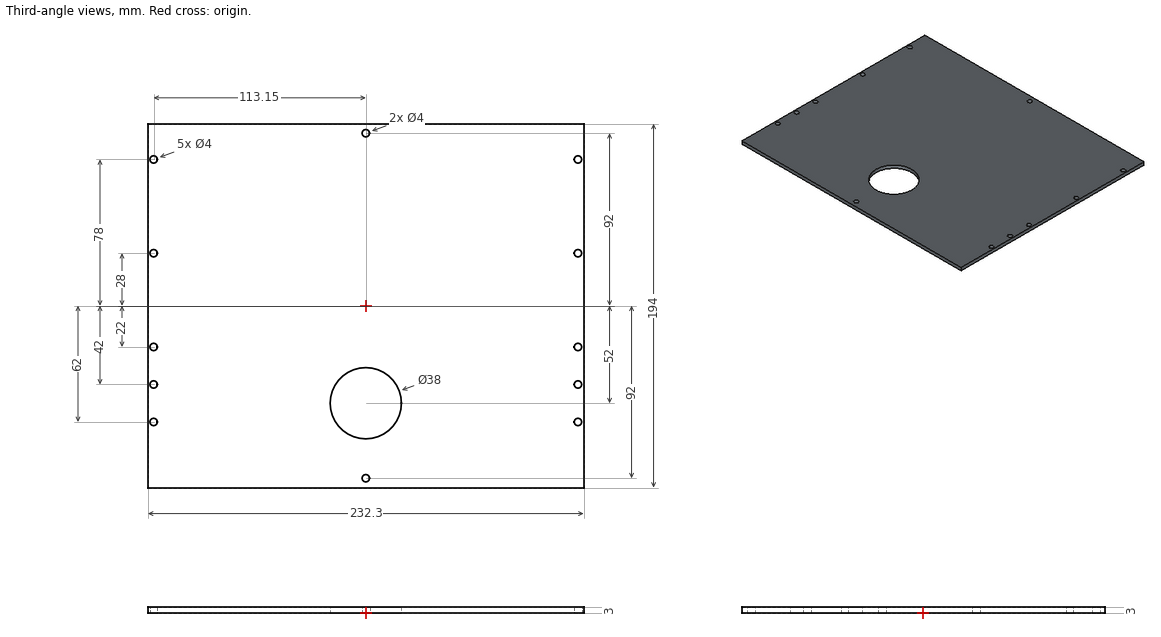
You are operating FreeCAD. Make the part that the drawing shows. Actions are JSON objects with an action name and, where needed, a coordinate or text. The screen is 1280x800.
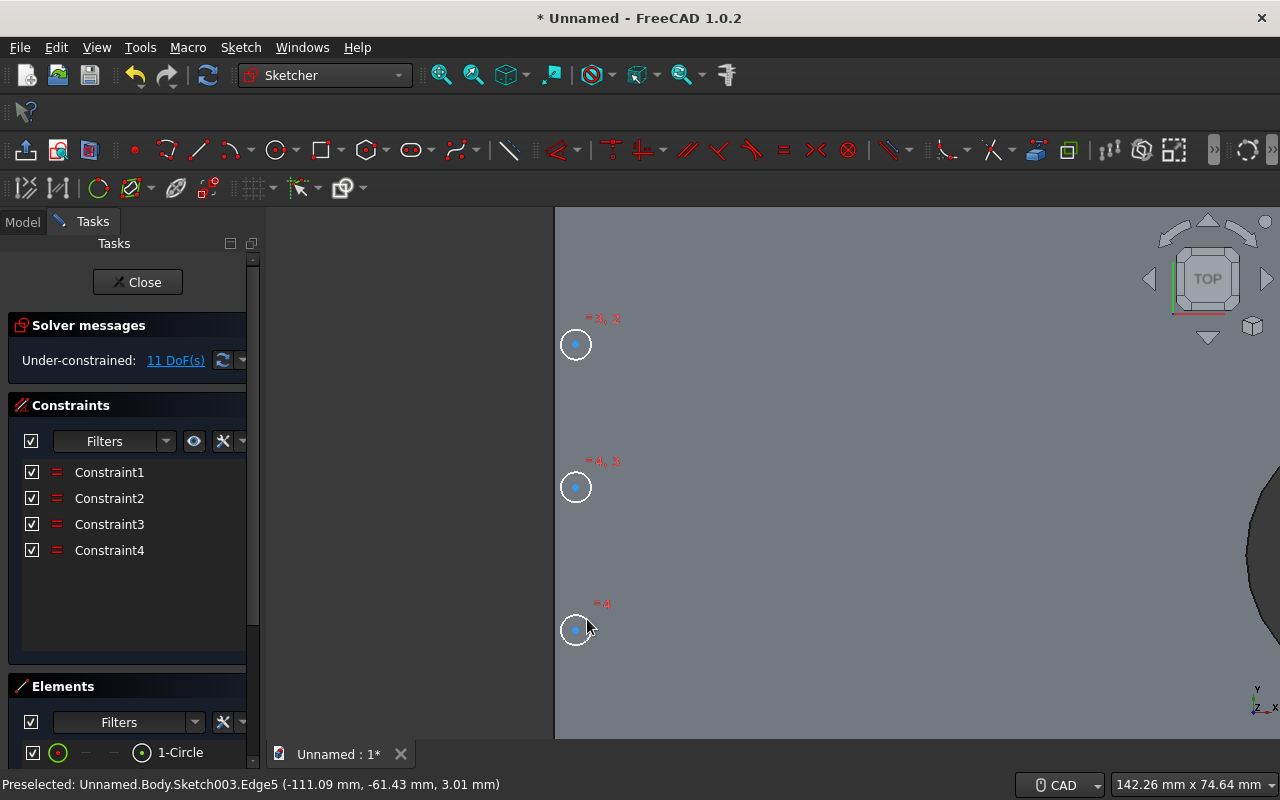
{"action": "scroll", "coordinate": [589, 622], "scroll_direction": "down", "scroll_amount": 6}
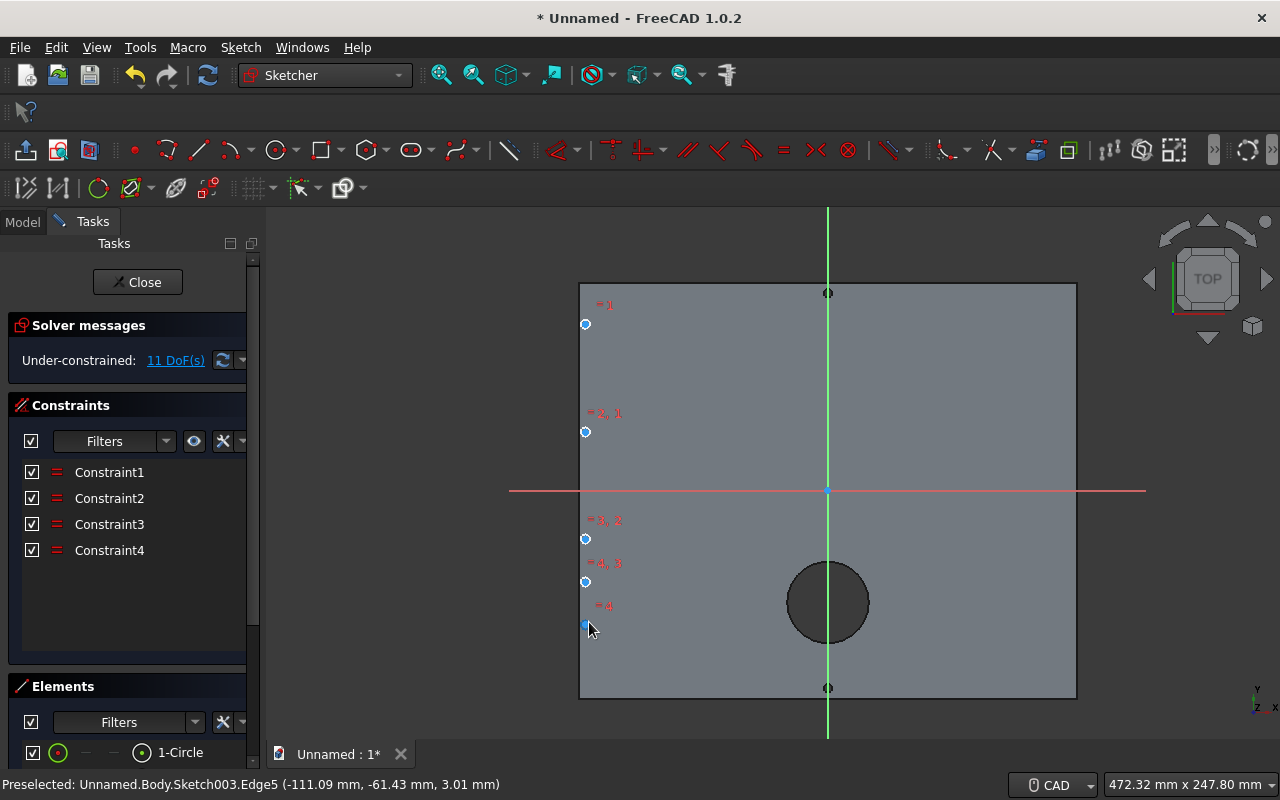
{"action": "left_click", "coordinate": [585, 324]}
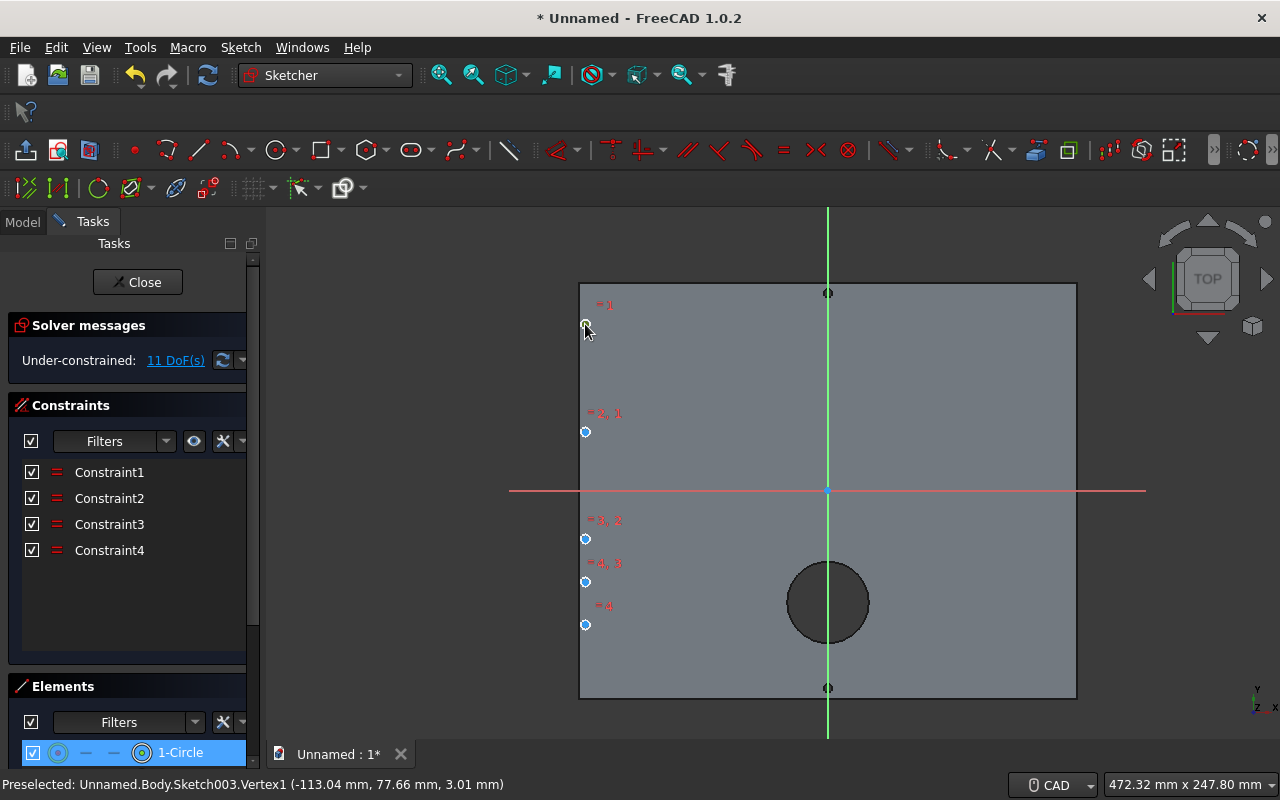
{"action": "left_click", "coordinate": [585, 432]}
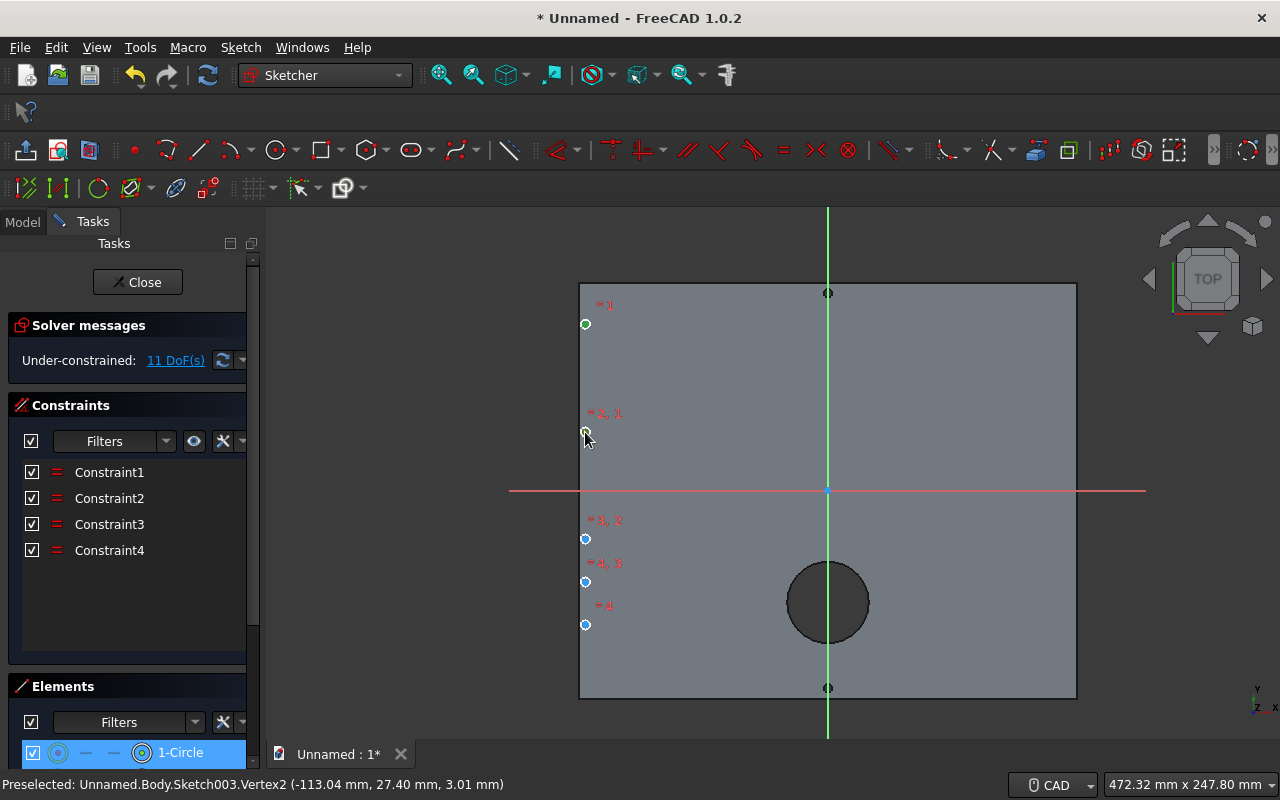
{"action": "key", "text": "v"}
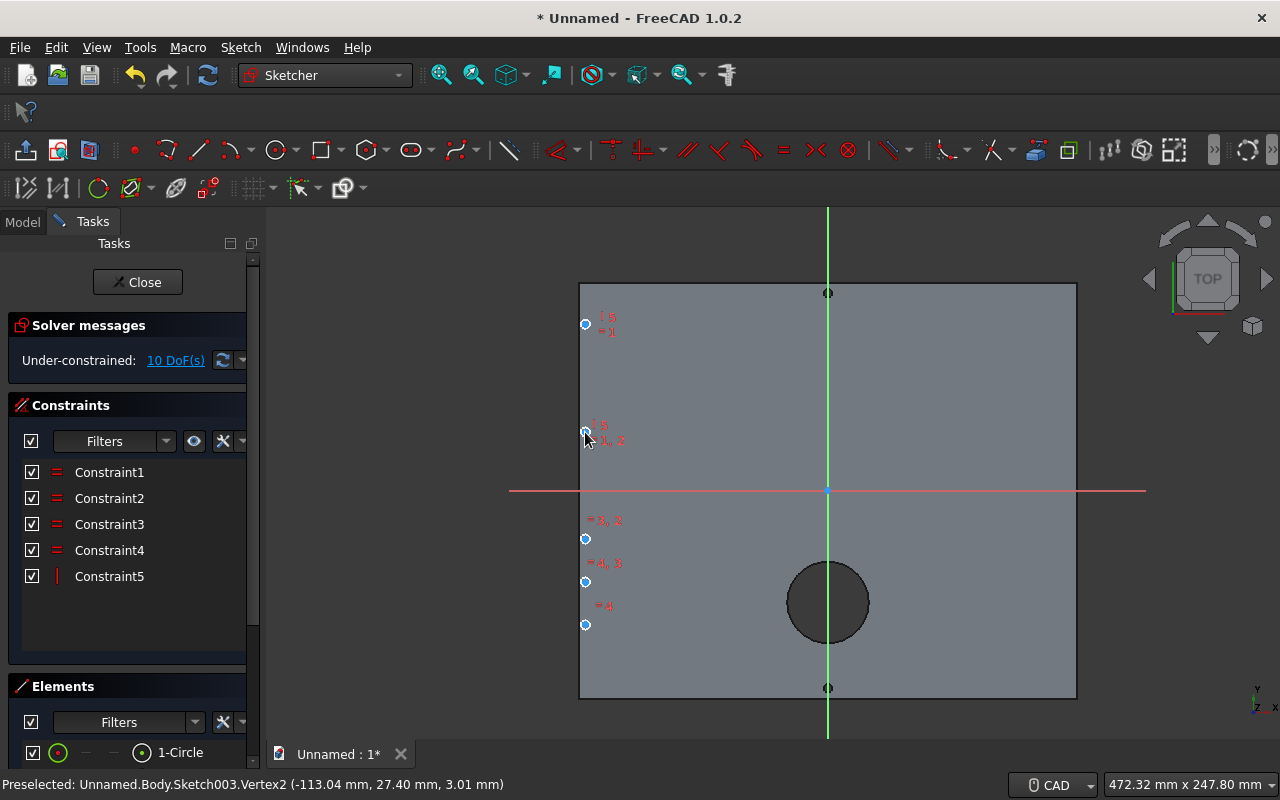
{"action": "left_click", "coordinate": [585, 432]}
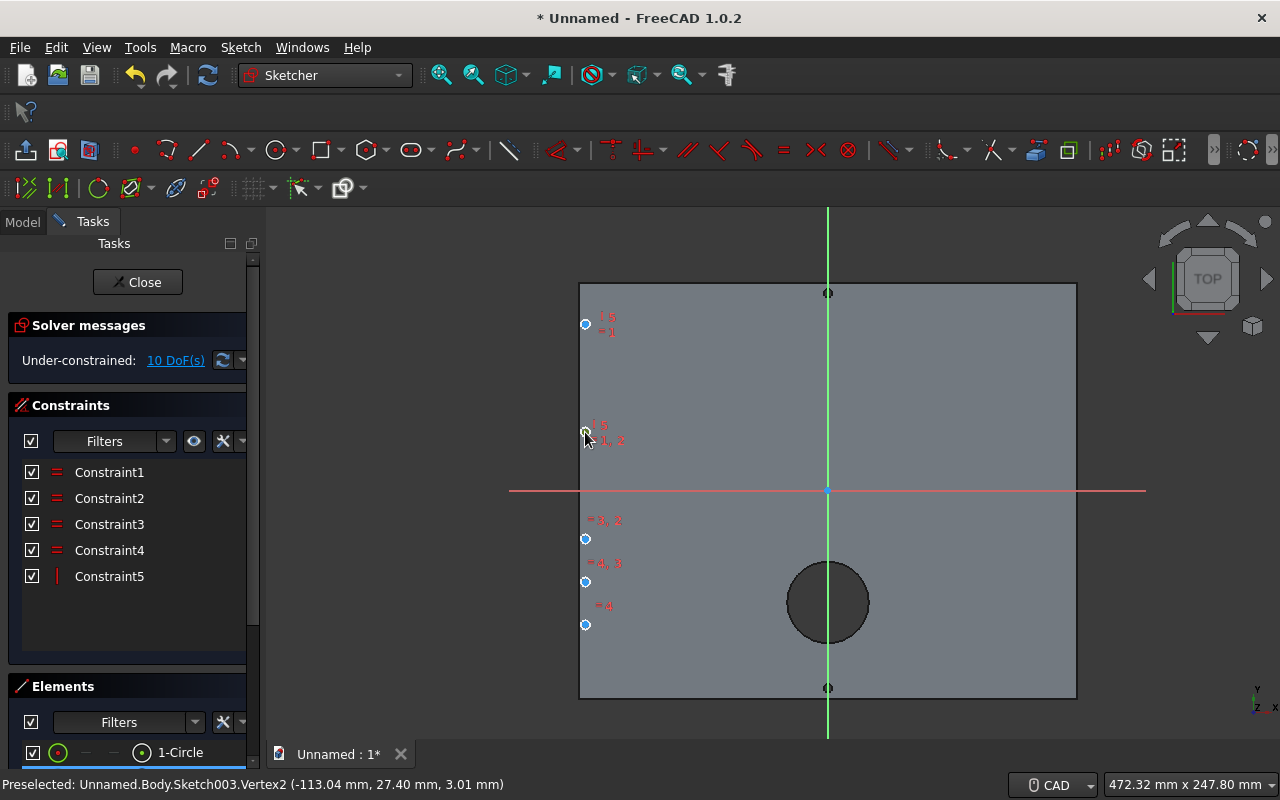
{"action": "left_click", "coordinate": [585, 539]}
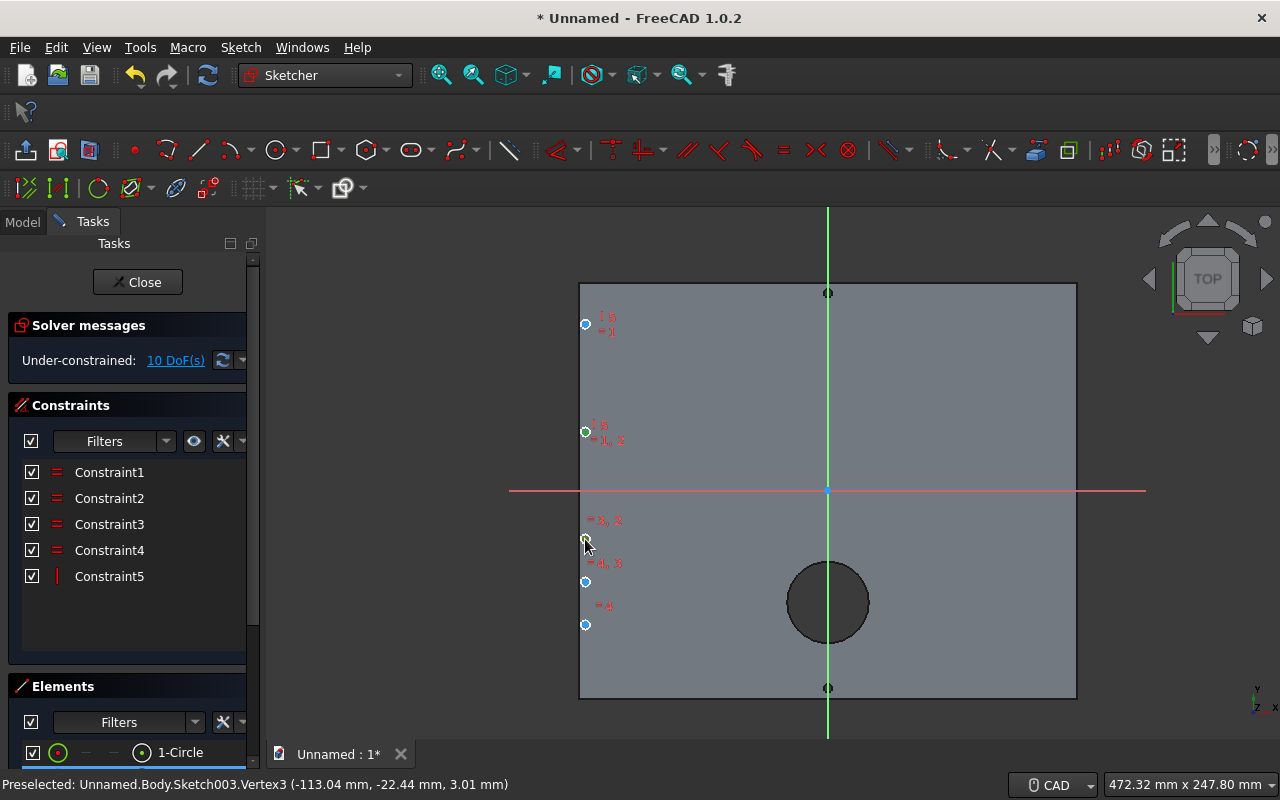
{"action": "key", "text": "v"}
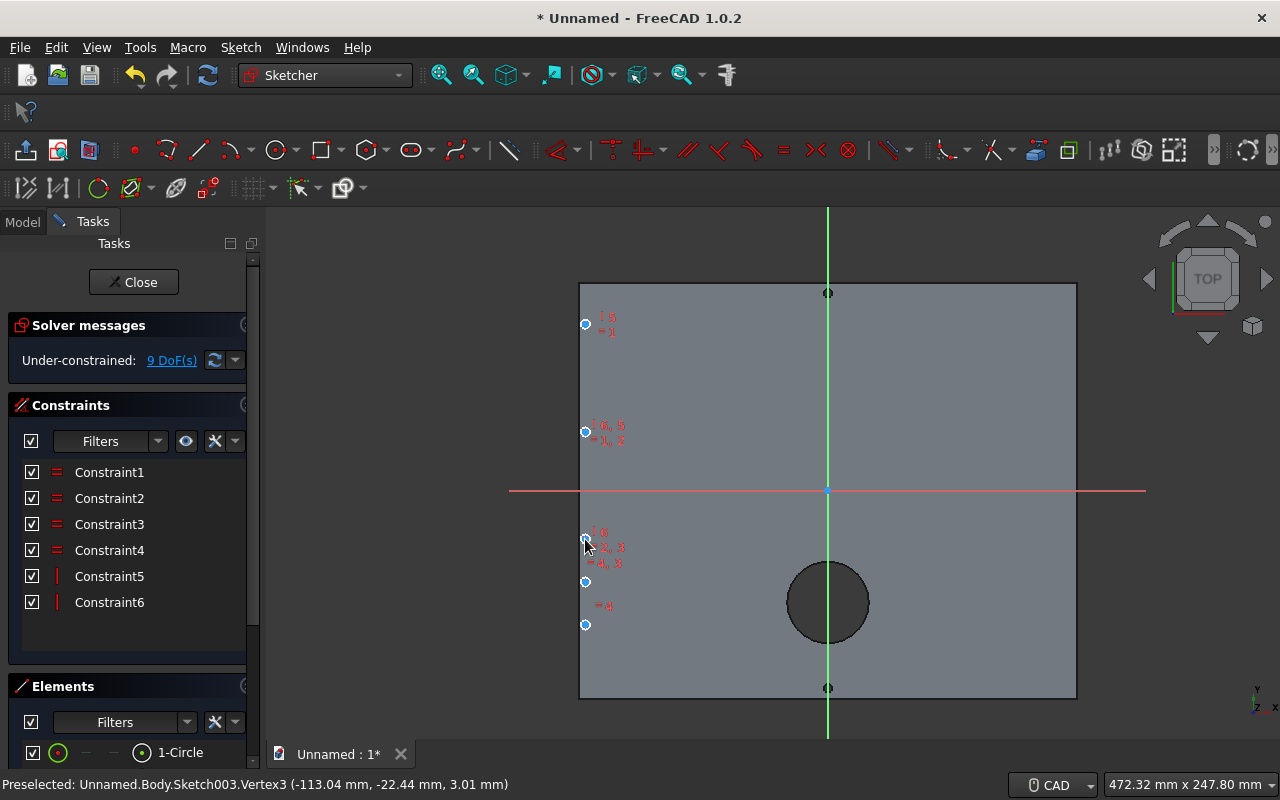
{"action": "left_click", "coordinate": [585, 539]}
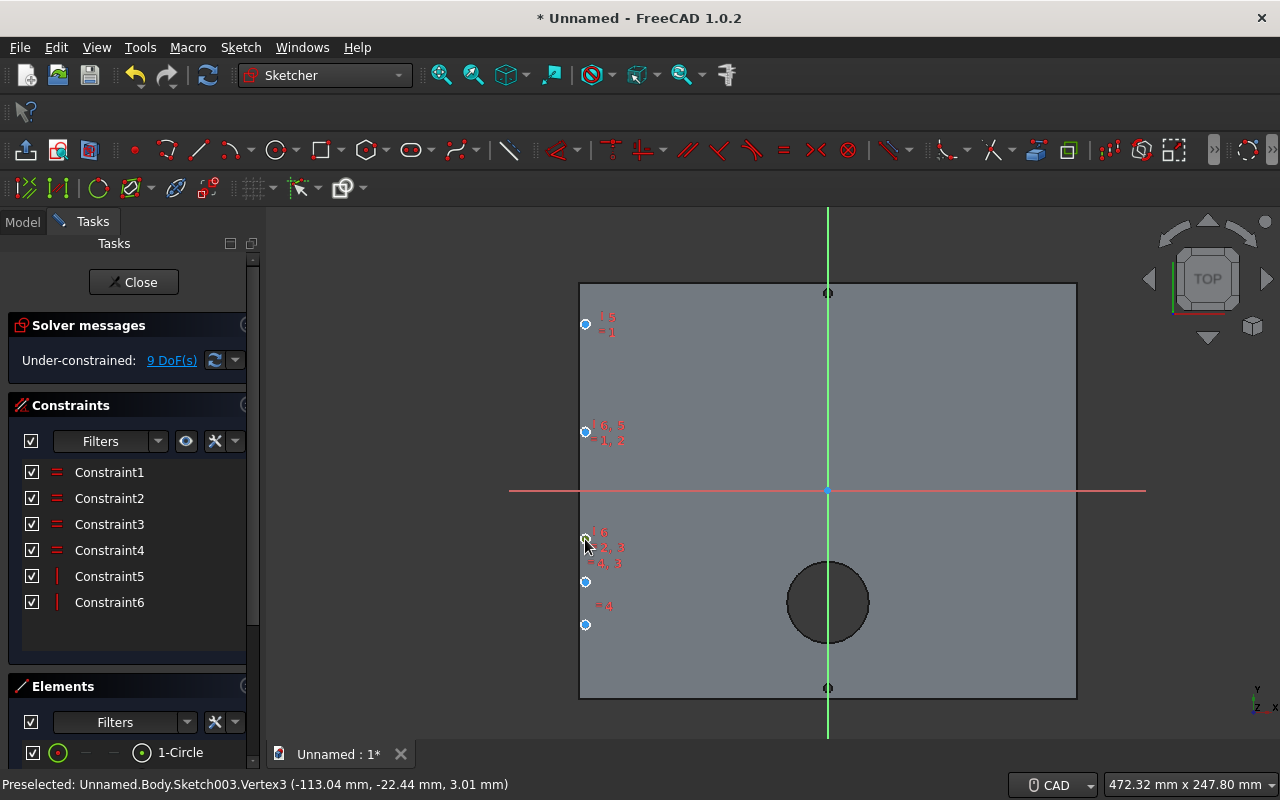
{"action": "left_click", "coordinate": [585, 582]}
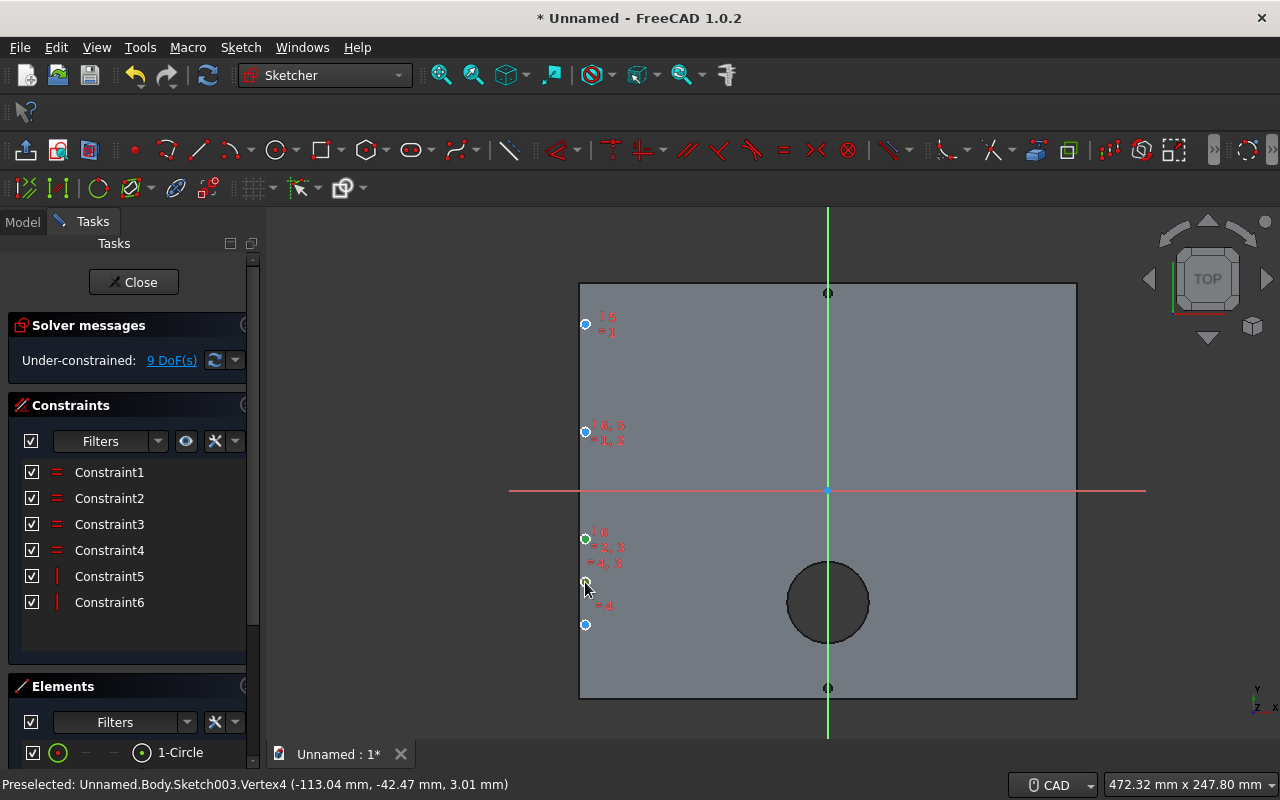
{"action": "key", "text": "v"}